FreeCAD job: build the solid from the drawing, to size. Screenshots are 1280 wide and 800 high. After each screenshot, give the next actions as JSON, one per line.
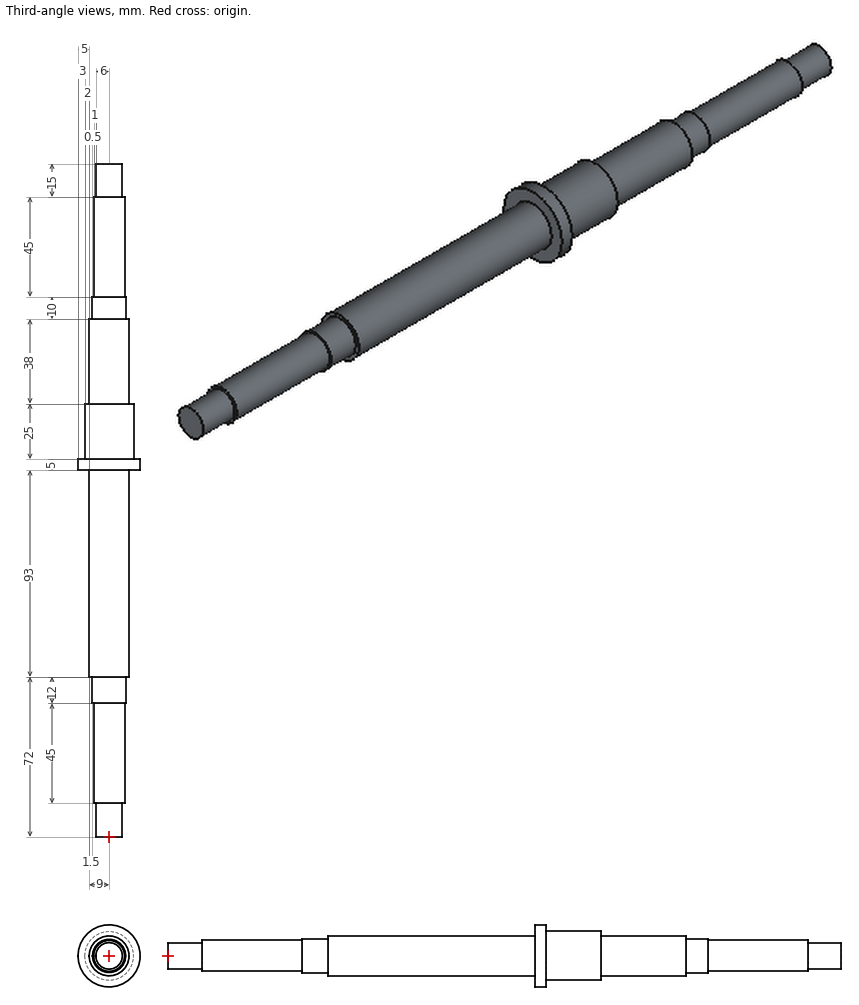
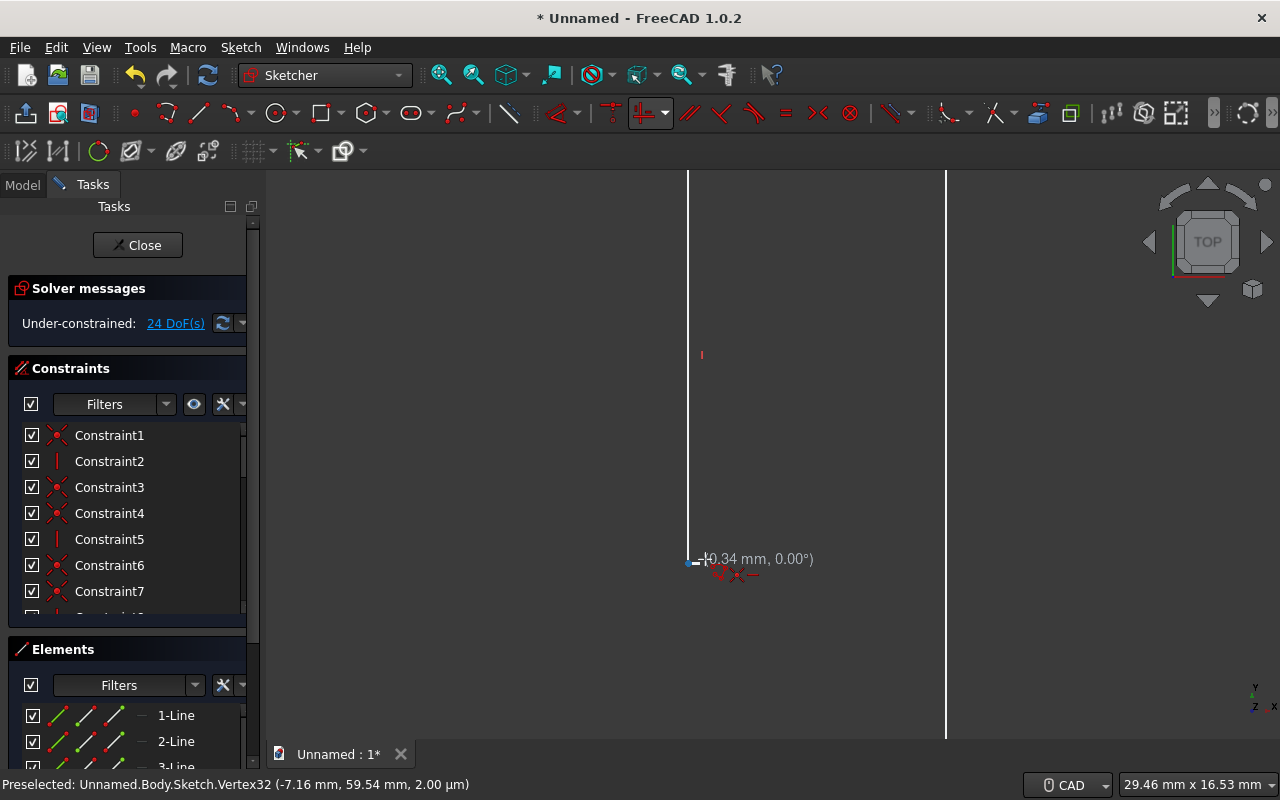
{"action": "left_click", "coordinate": [705, 550]}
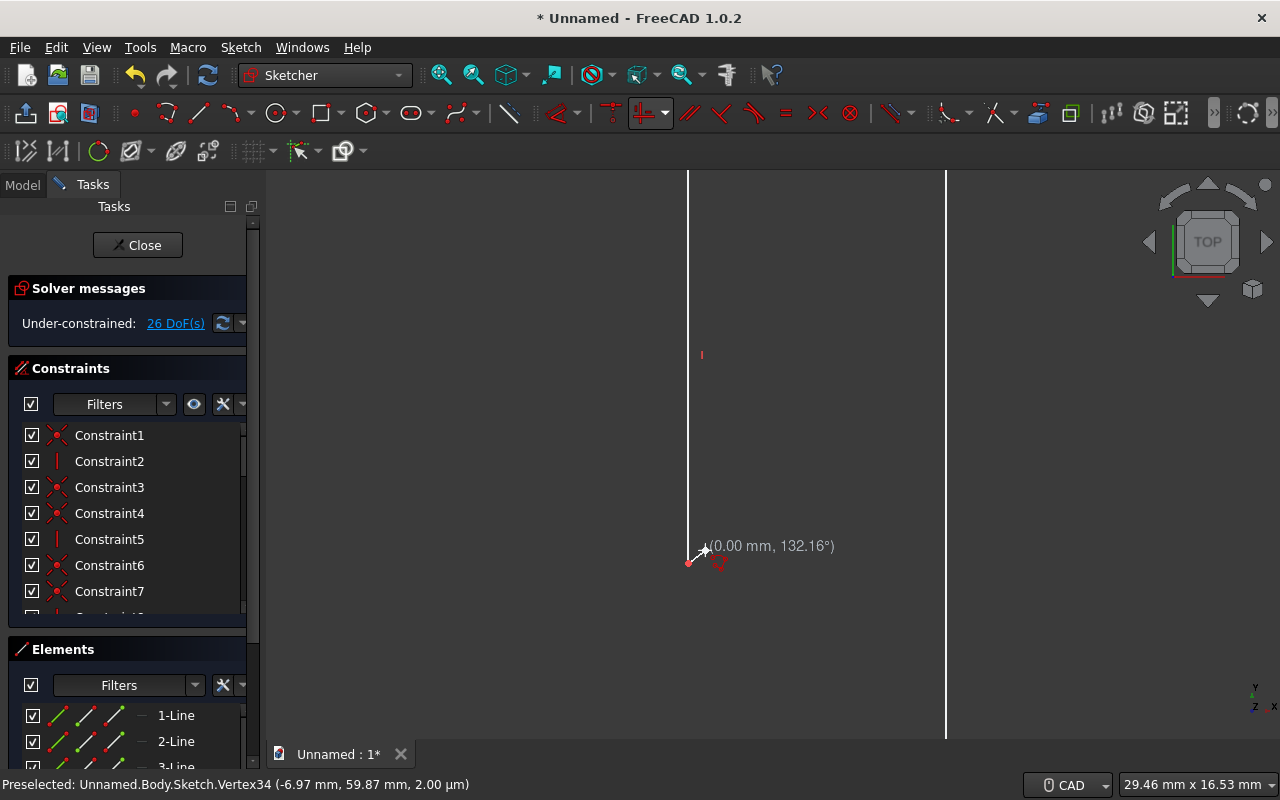
{"action": "scroll", "coordinate": [704, 584], "scroll_direction": "down", "scroll_amount": 16}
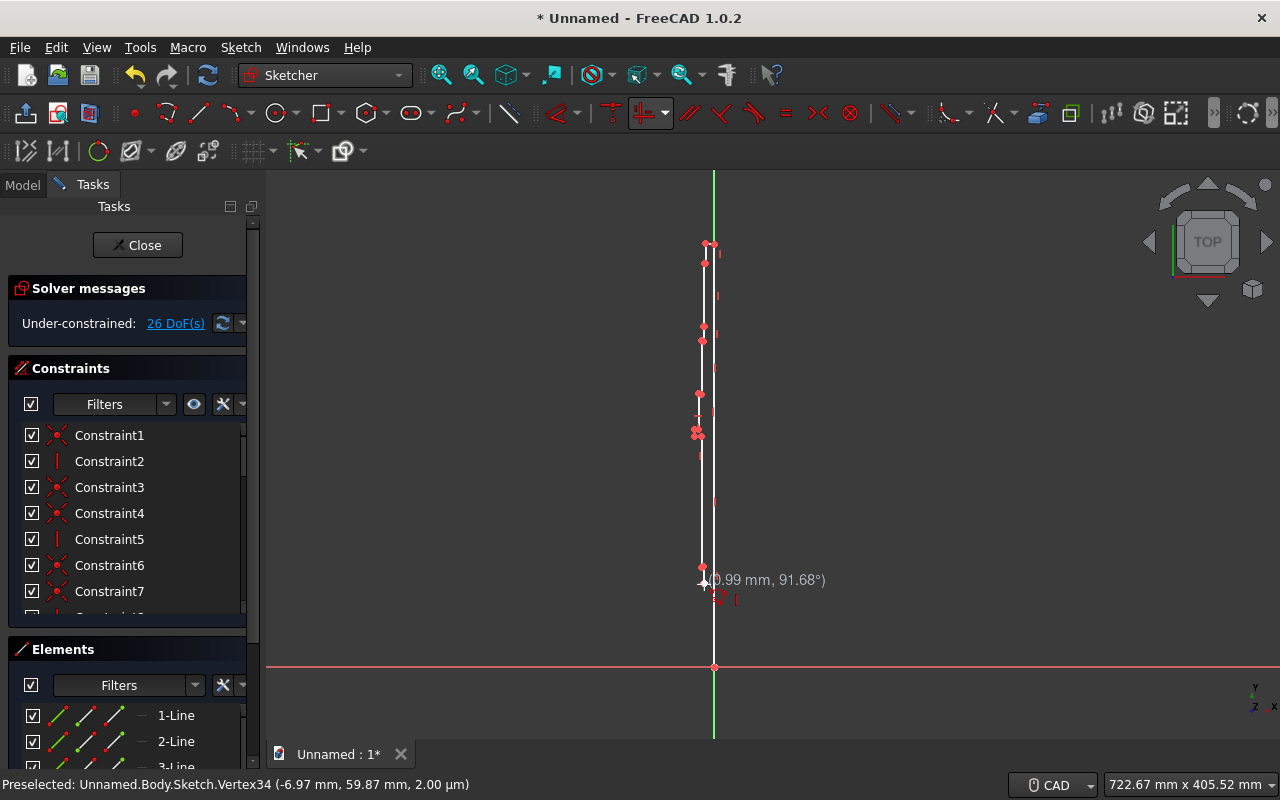
{"action": "scroll", "coordinate": [704, 646], "scroll_direction": "up", "scroll_amount": 3}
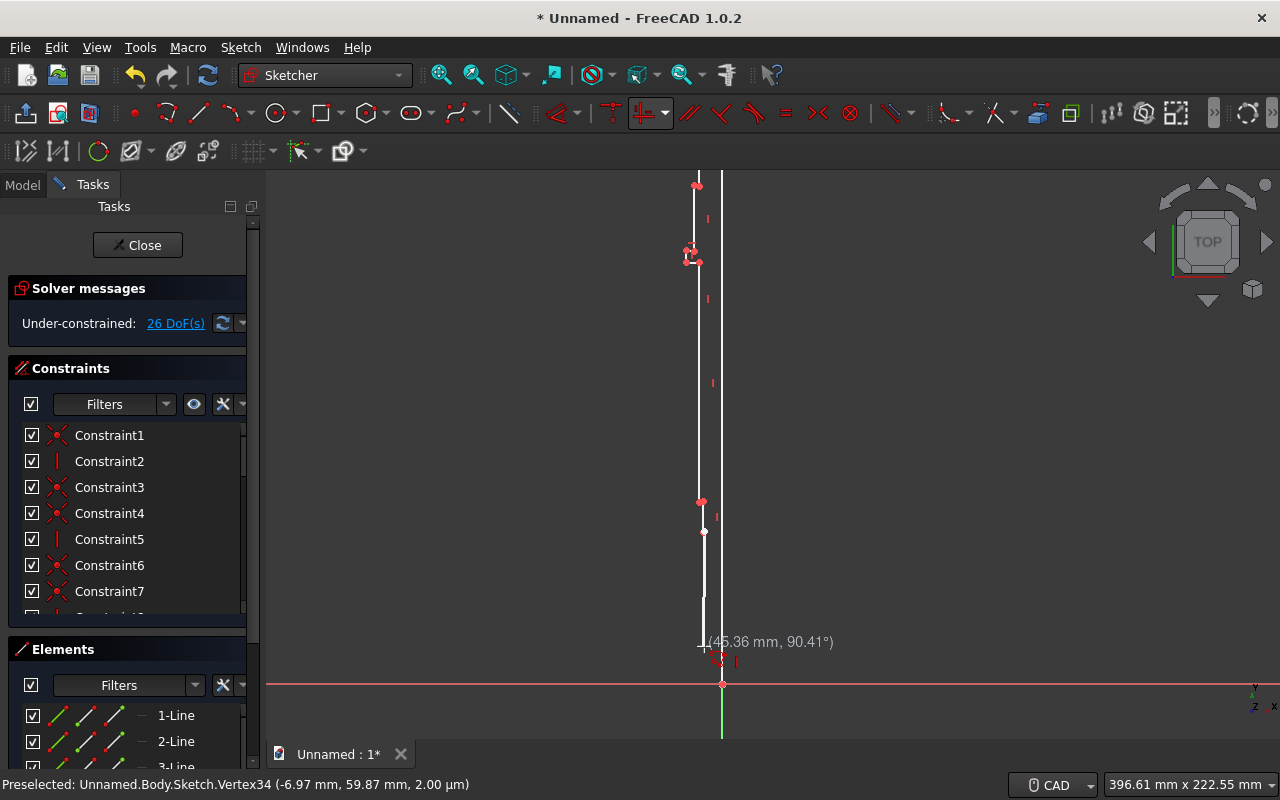
{"action": "left_click", "coordinate": [704, 646]}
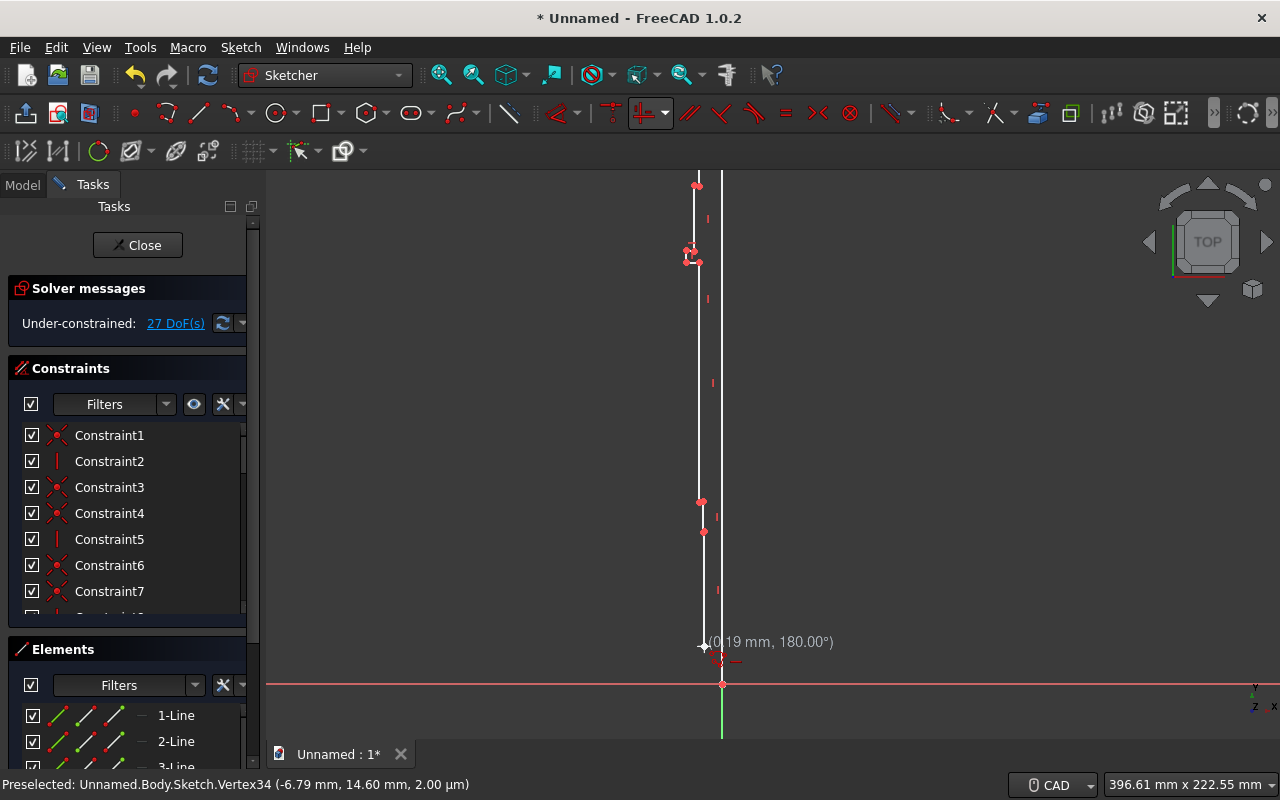
{"action": "scroll", "coordinate": [707, 646], "scroll_direction": "up", "scroll_amount": 10}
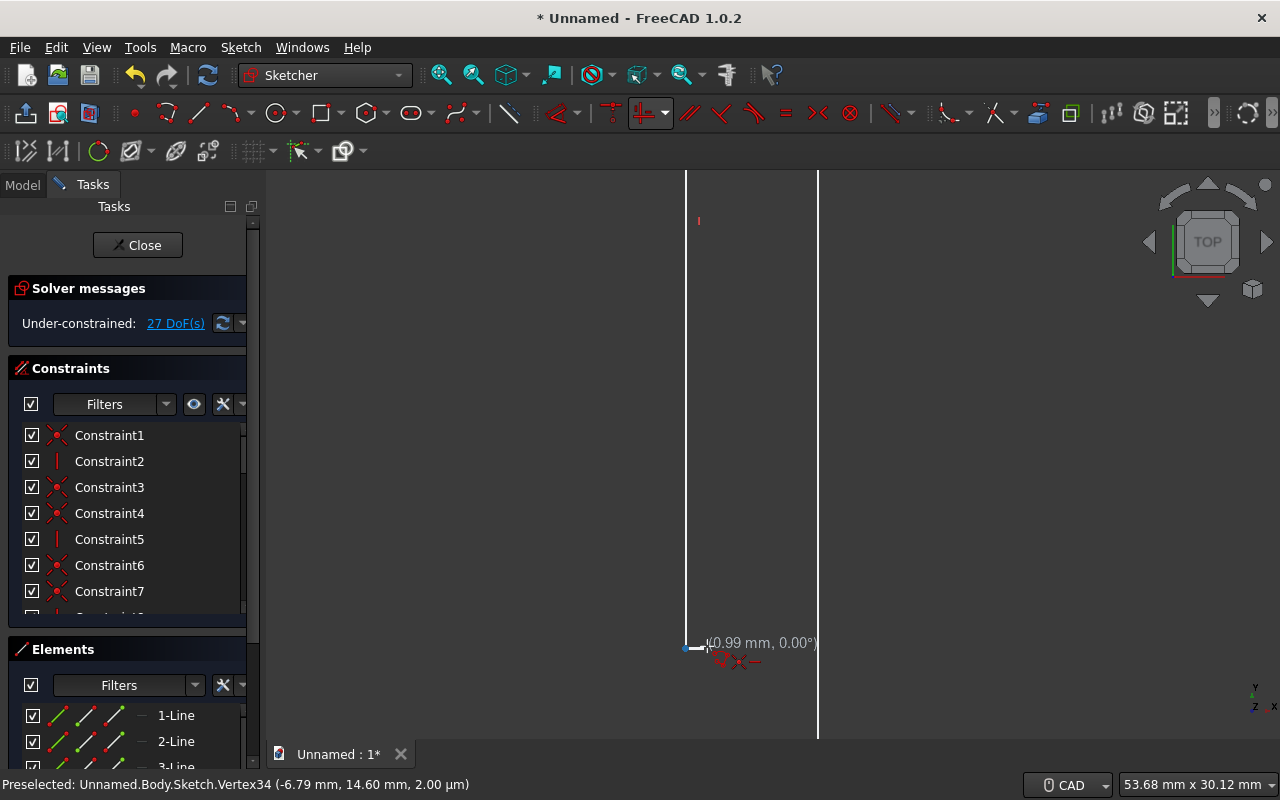
{"action": "left_click", "coordinate": [704, 641]}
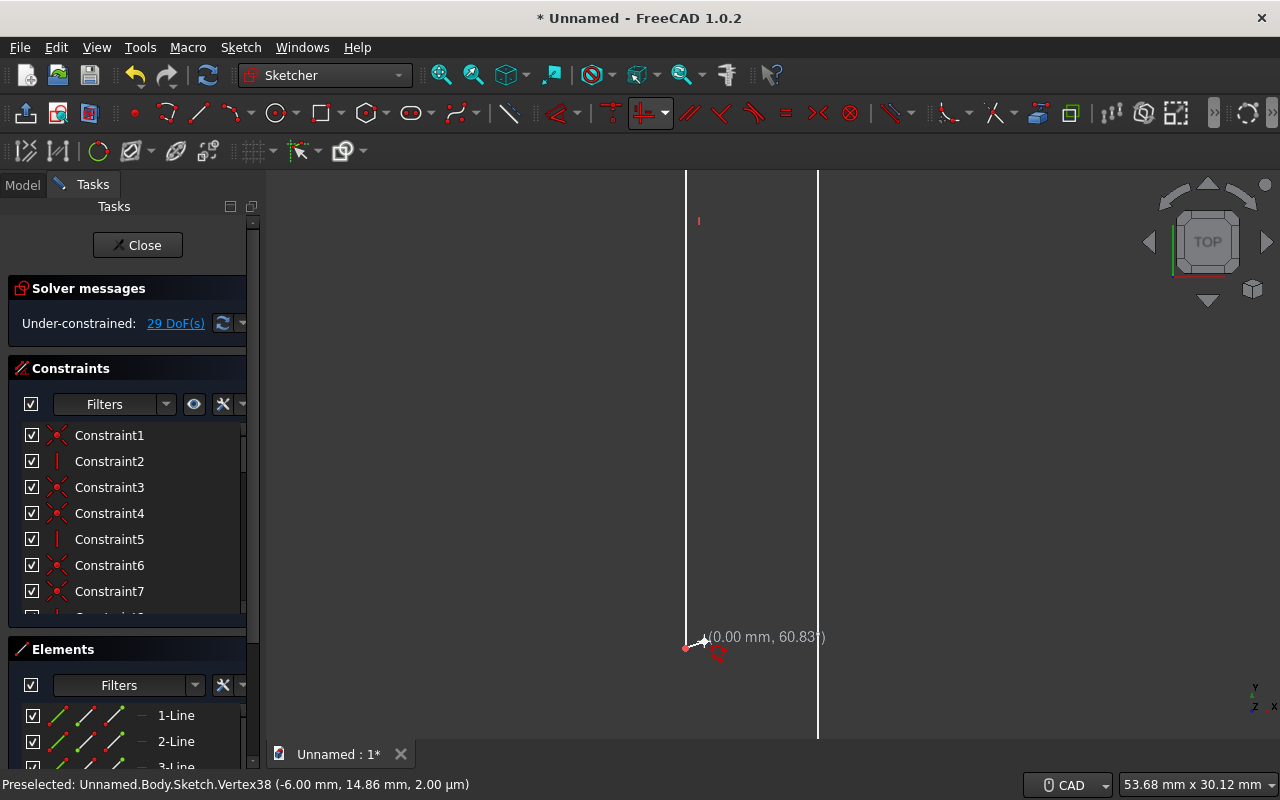
{"action": "scroll", "coordinate": [706, 609], "scroll_direction": "down", "scroll_amount": 14}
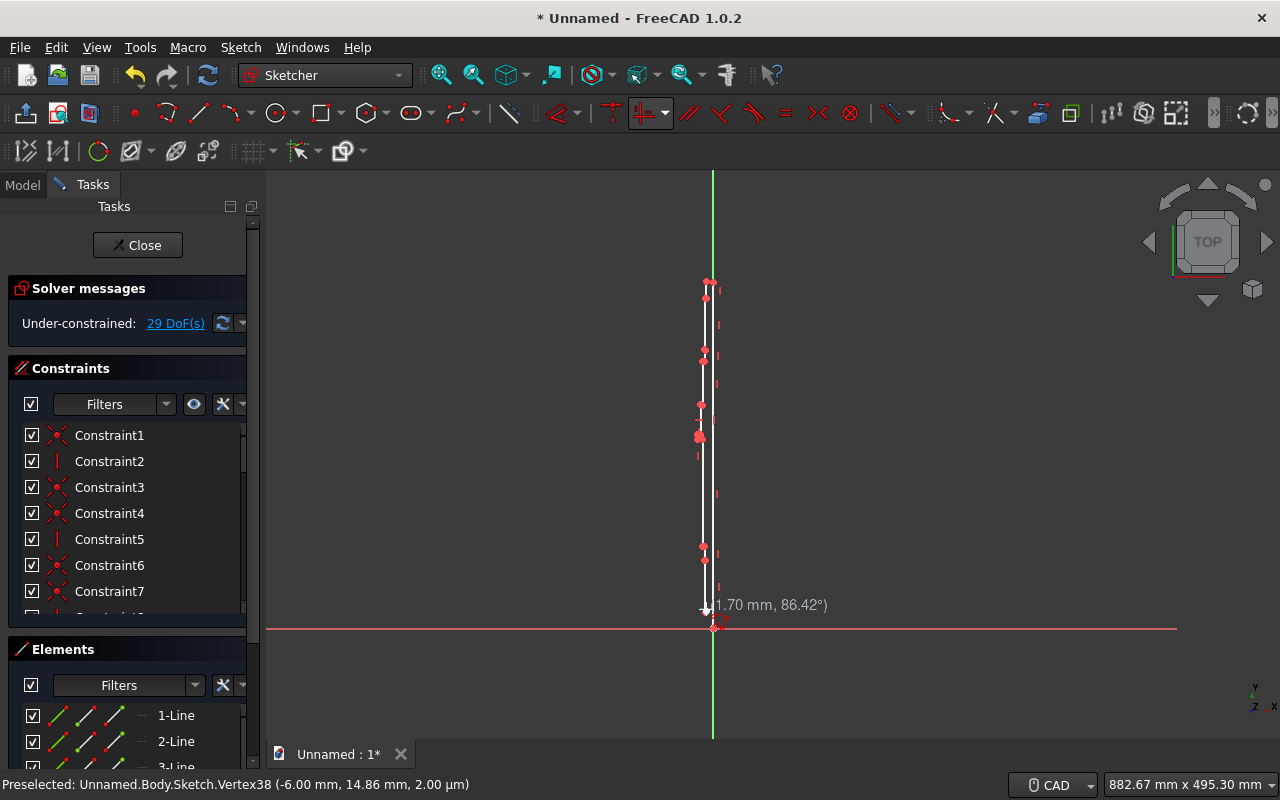
{"action": "scroll", "coordinate": [706, 629], "scroll_direction": "up", "scroll_amount": 5}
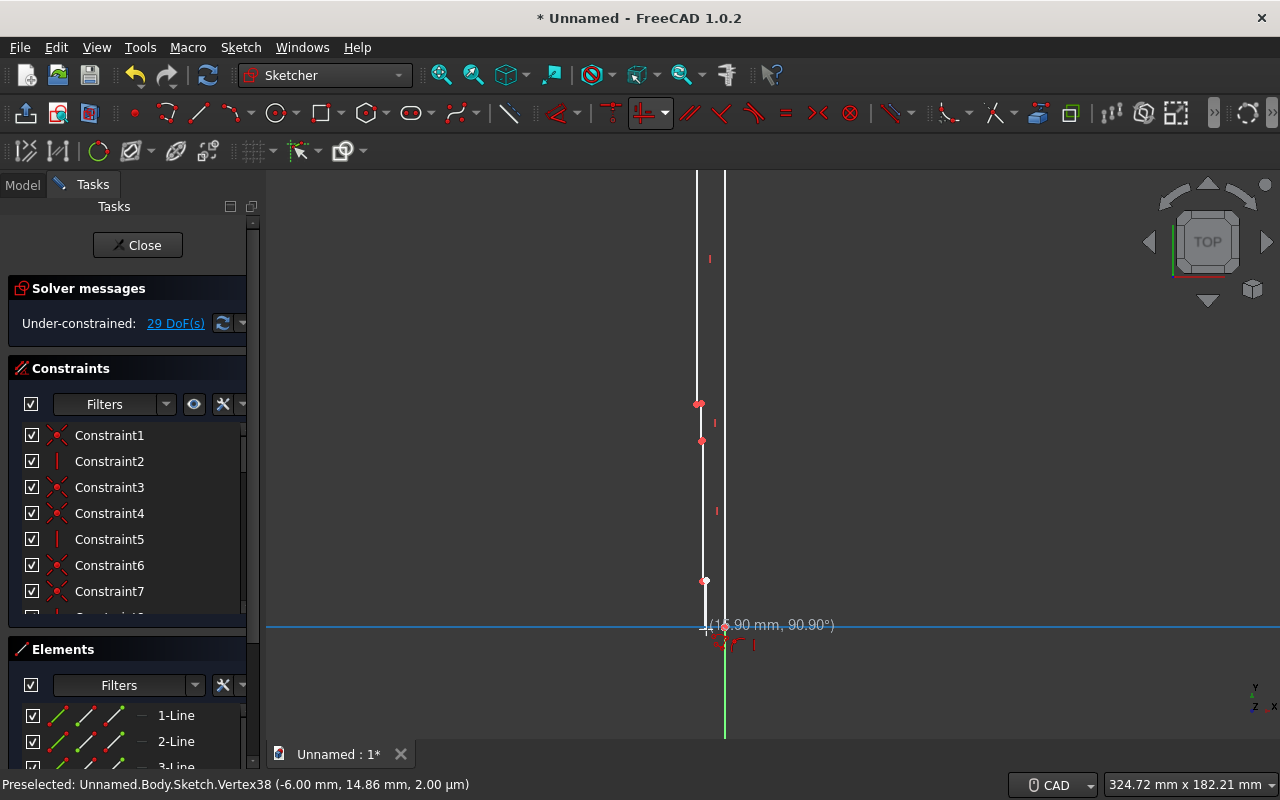
{"action": "left_click", "coordinate": [706, 618]}
{"action": "left_click", "coordinate": [725, 627]}
{"action": "key", "text": "Escape"}
{"action": "key", "text": "Escape"}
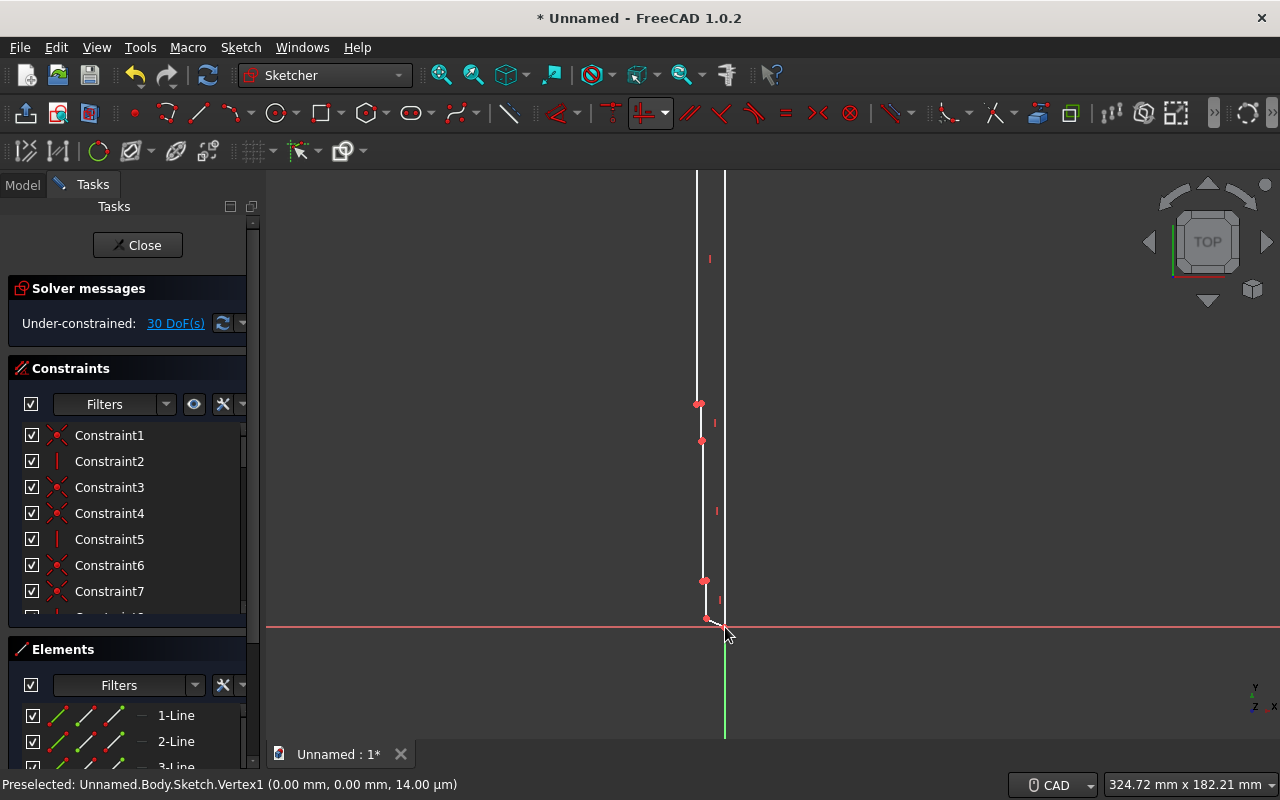
{"action": "scroll", "coordinate": [705, 629], "scroll_direction": "down", "scroll_amount": 5}